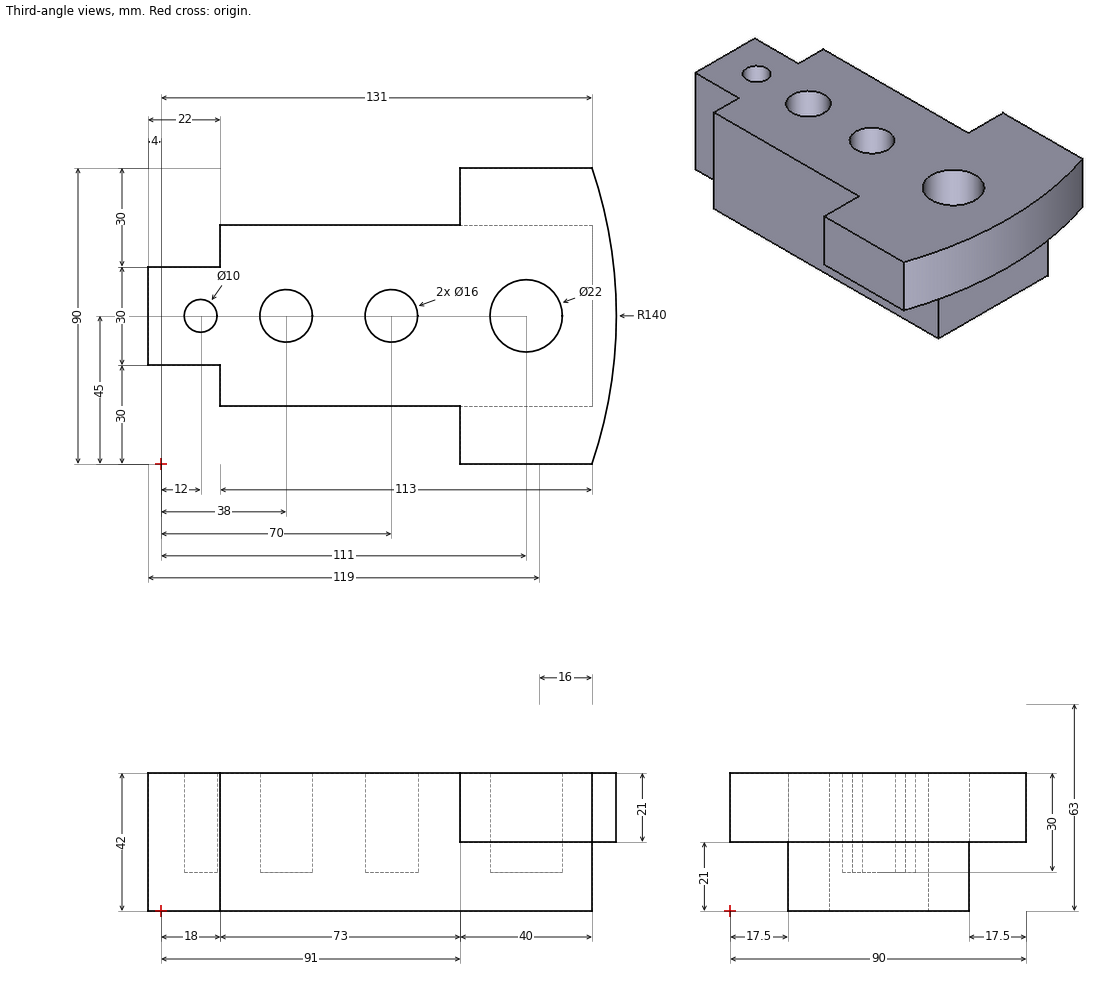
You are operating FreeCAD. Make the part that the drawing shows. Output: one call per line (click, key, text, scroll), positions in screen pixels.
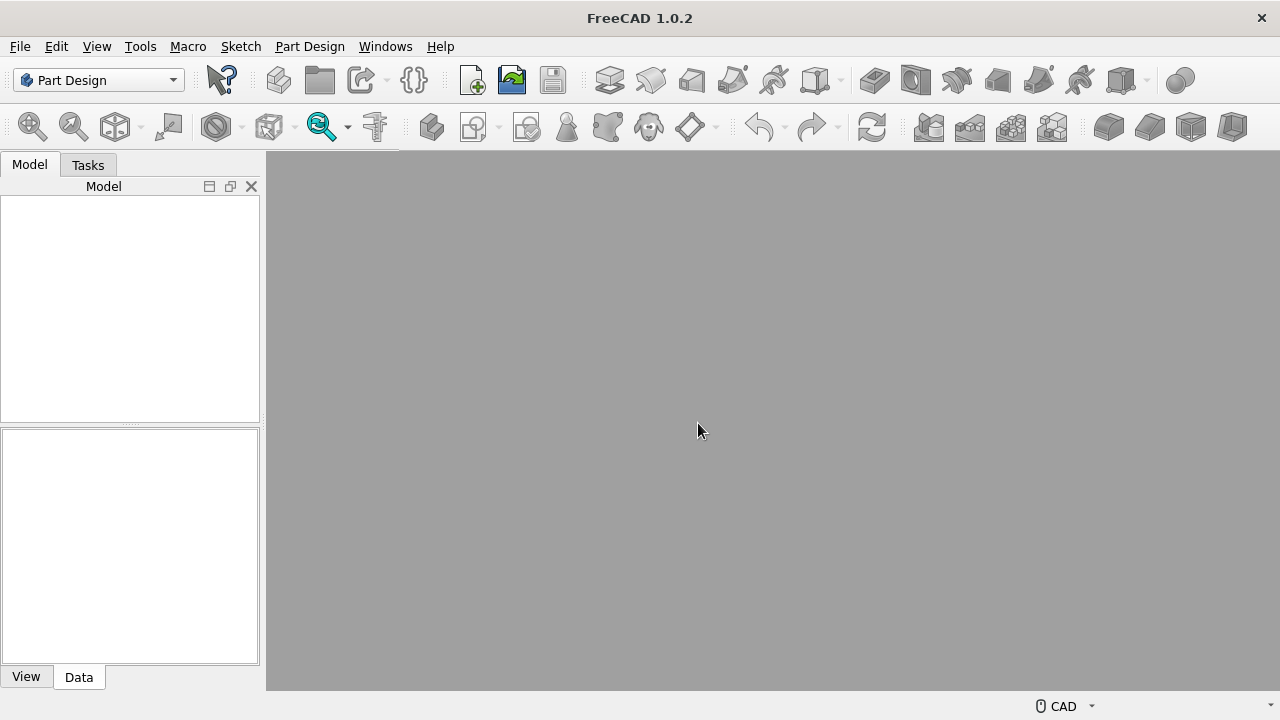
click(471, 80)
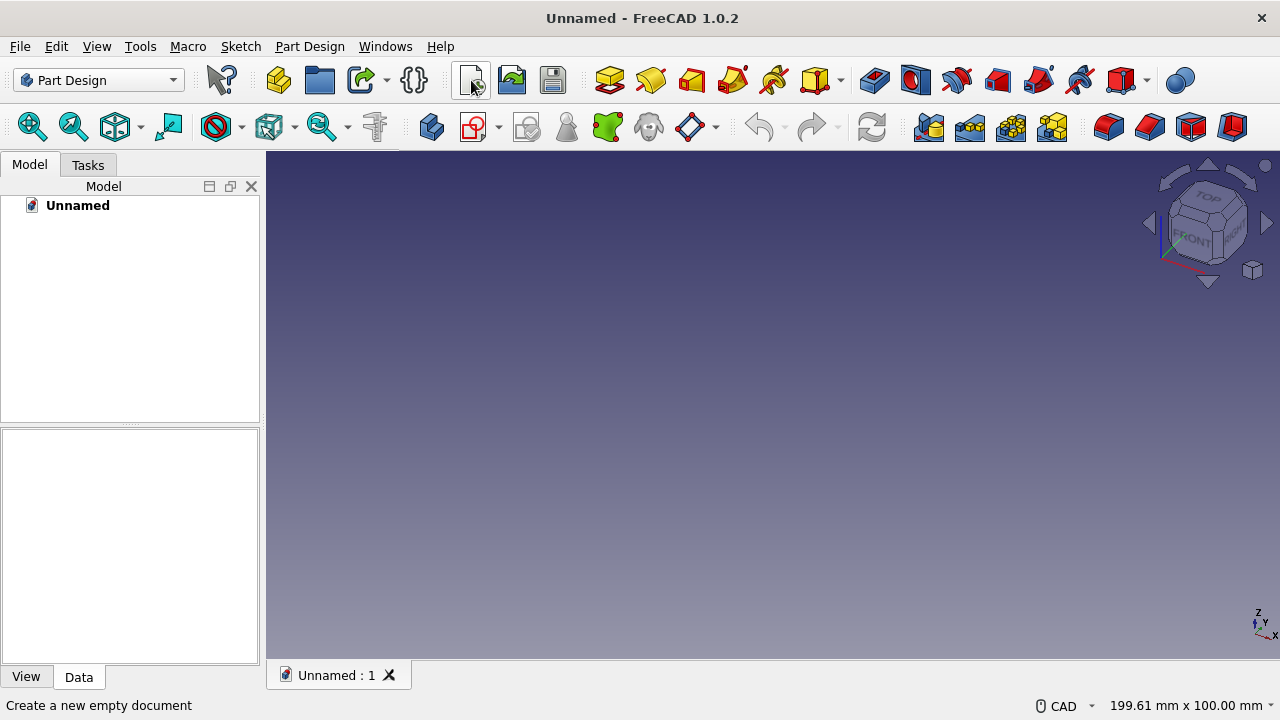
click(472, 128)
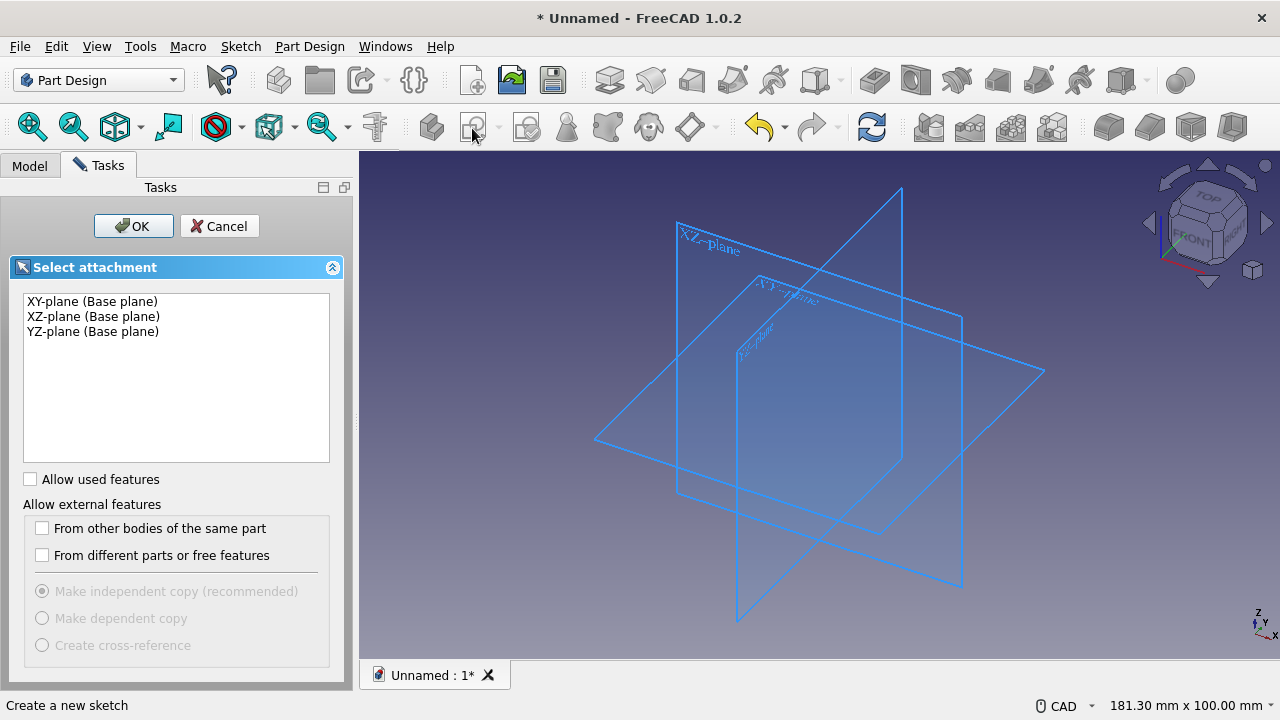
click(84, 302)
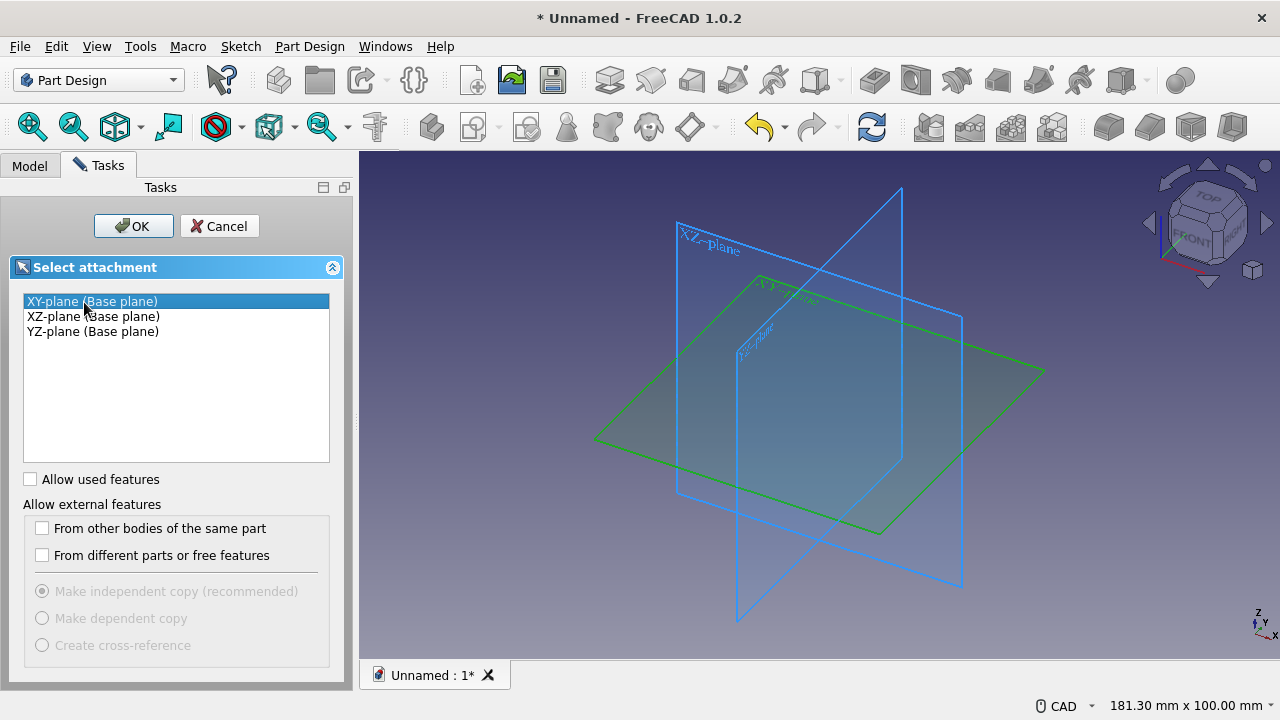
click(134, 226)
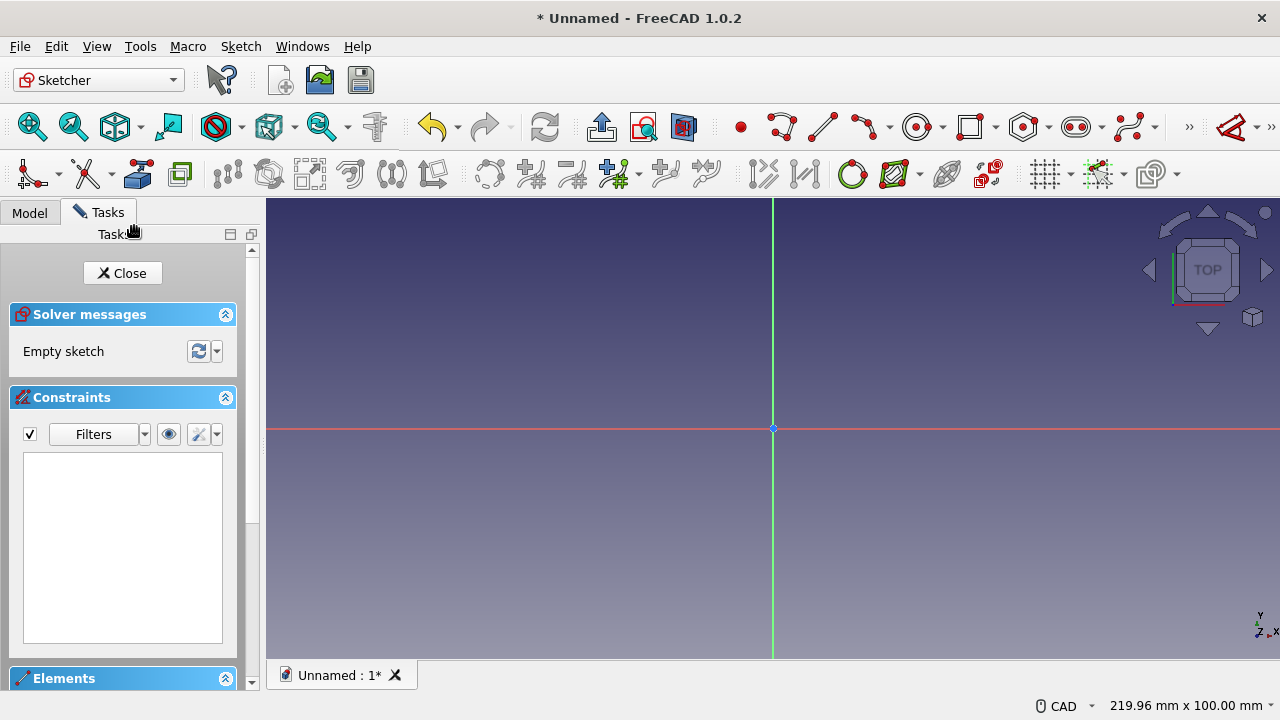
scroll(310, 631, down, 3)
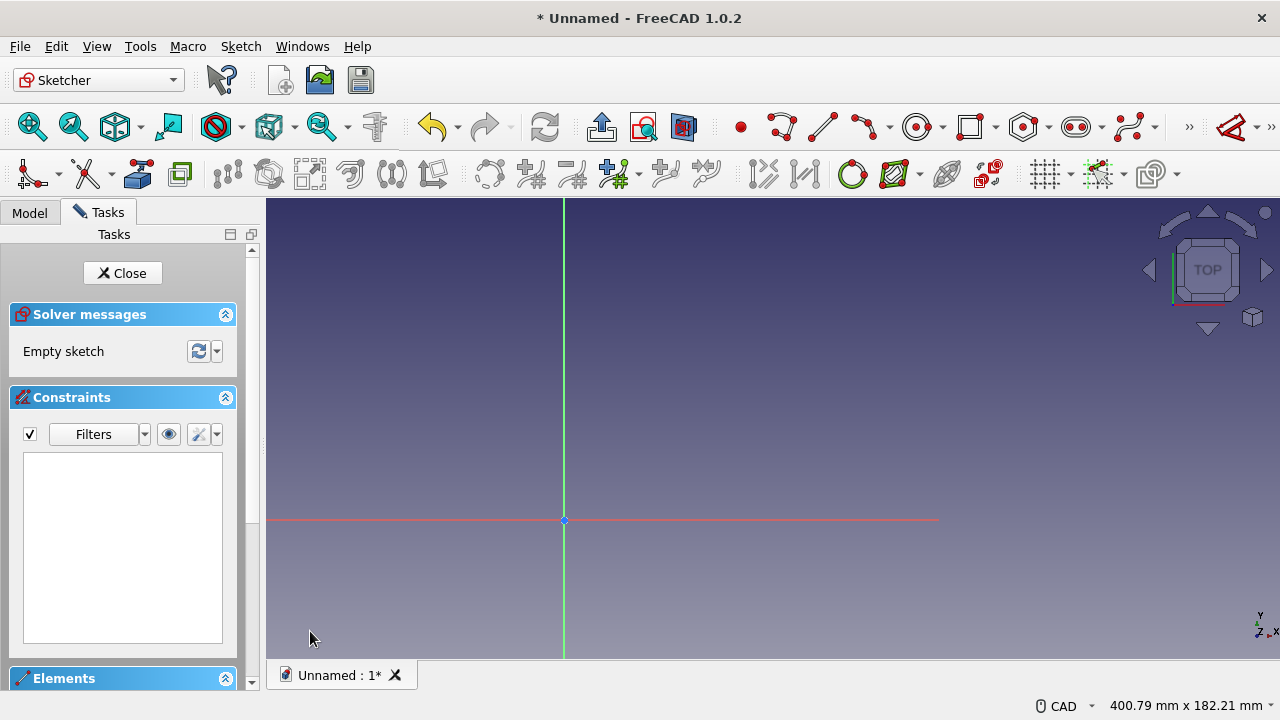
click(970, 128)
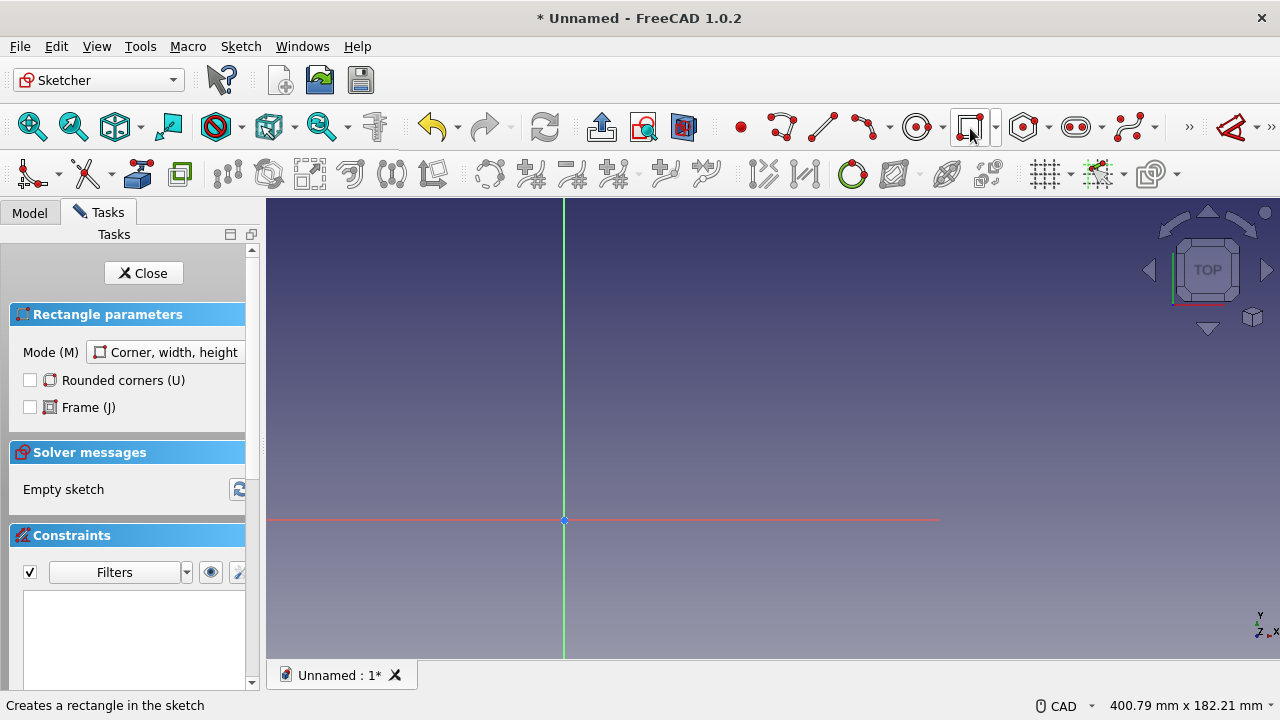
scroll(554, 293, up, 3)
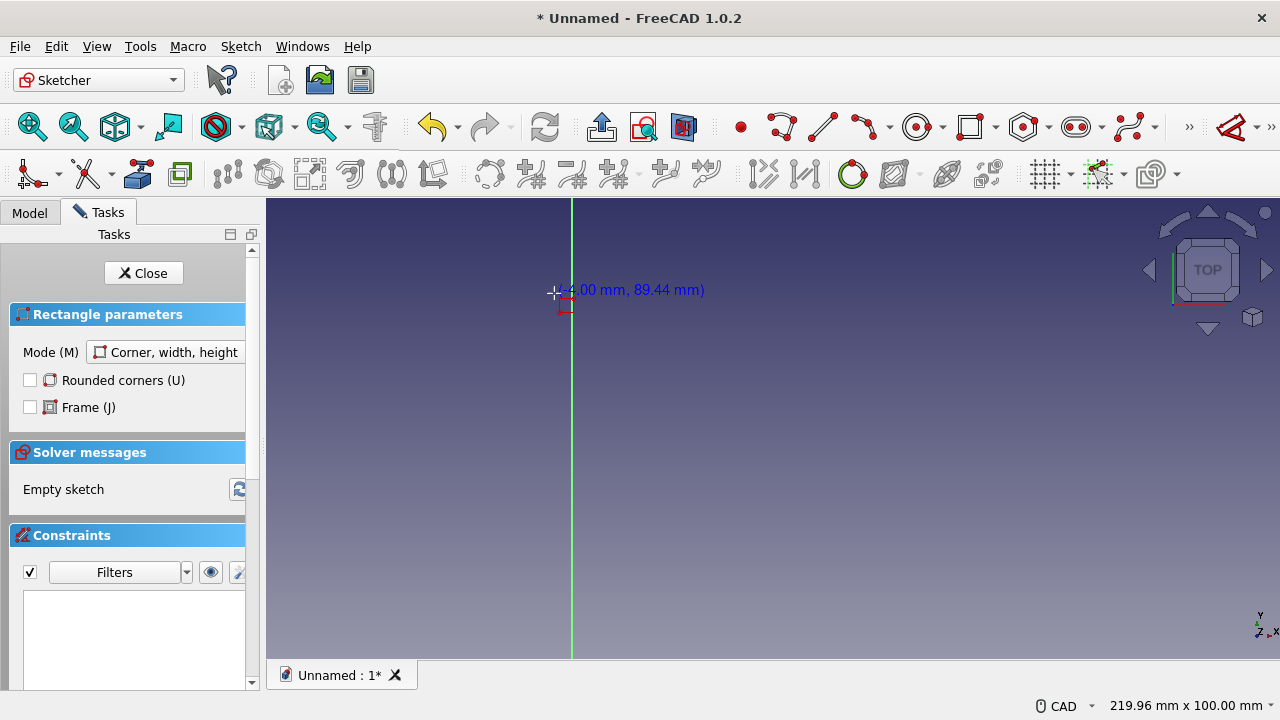
click(554, 292)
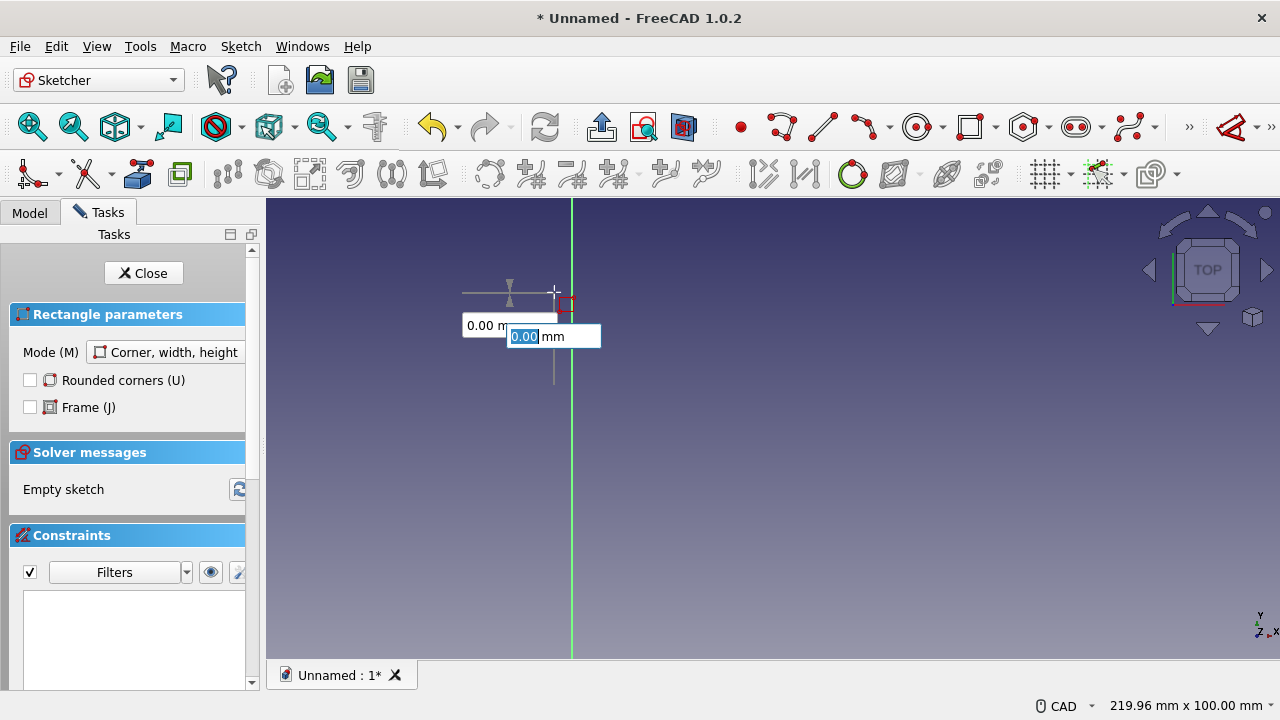
scroll(453, 284, down, 2)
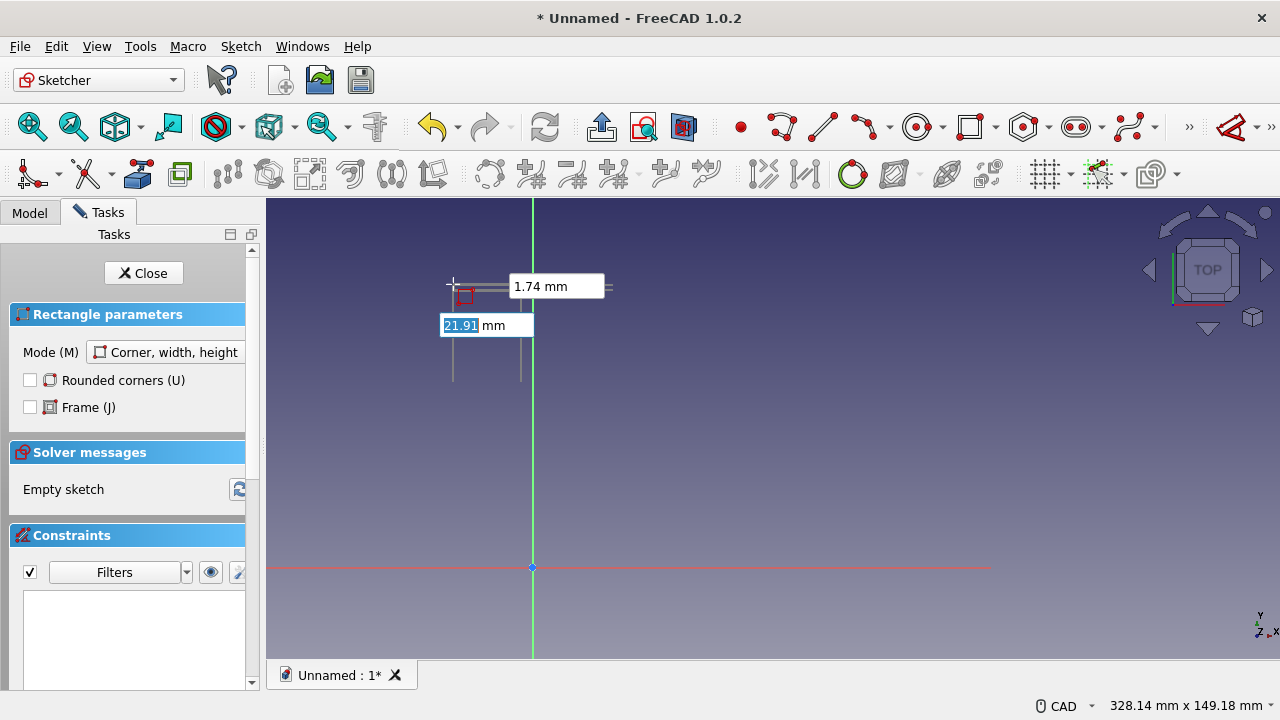
click(888, 568)
key(Escape)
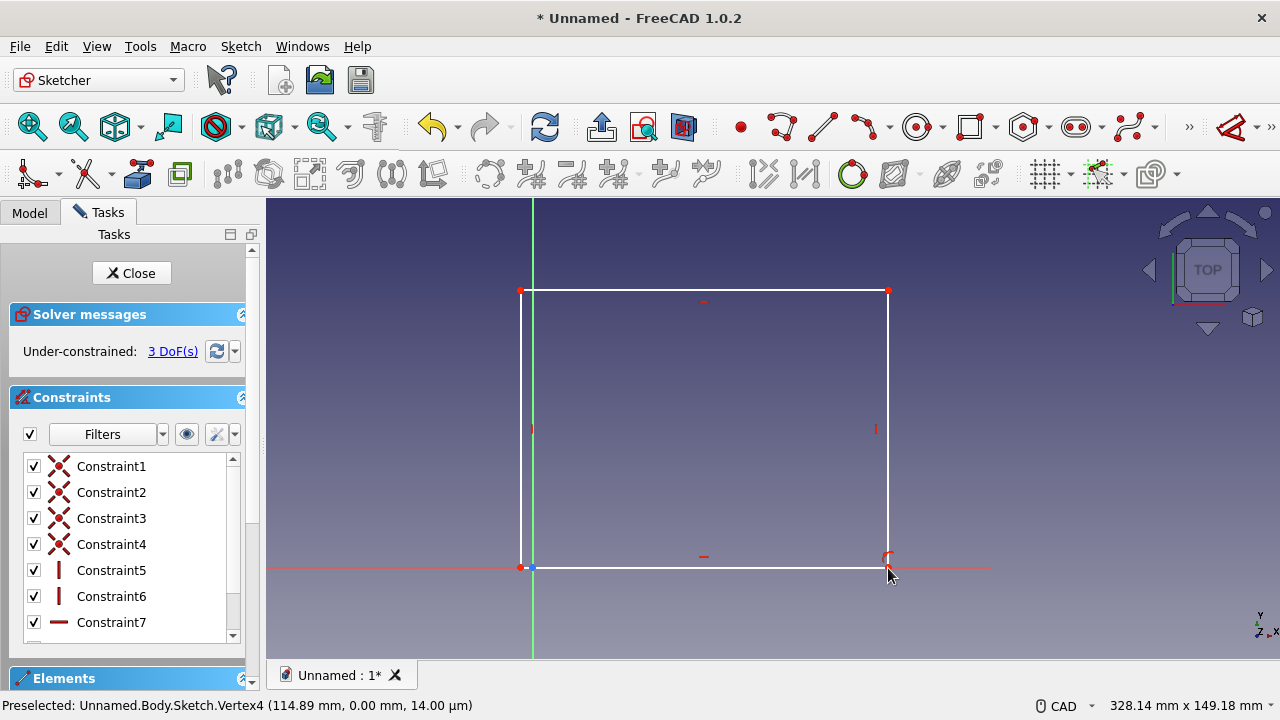
click(521, 373)